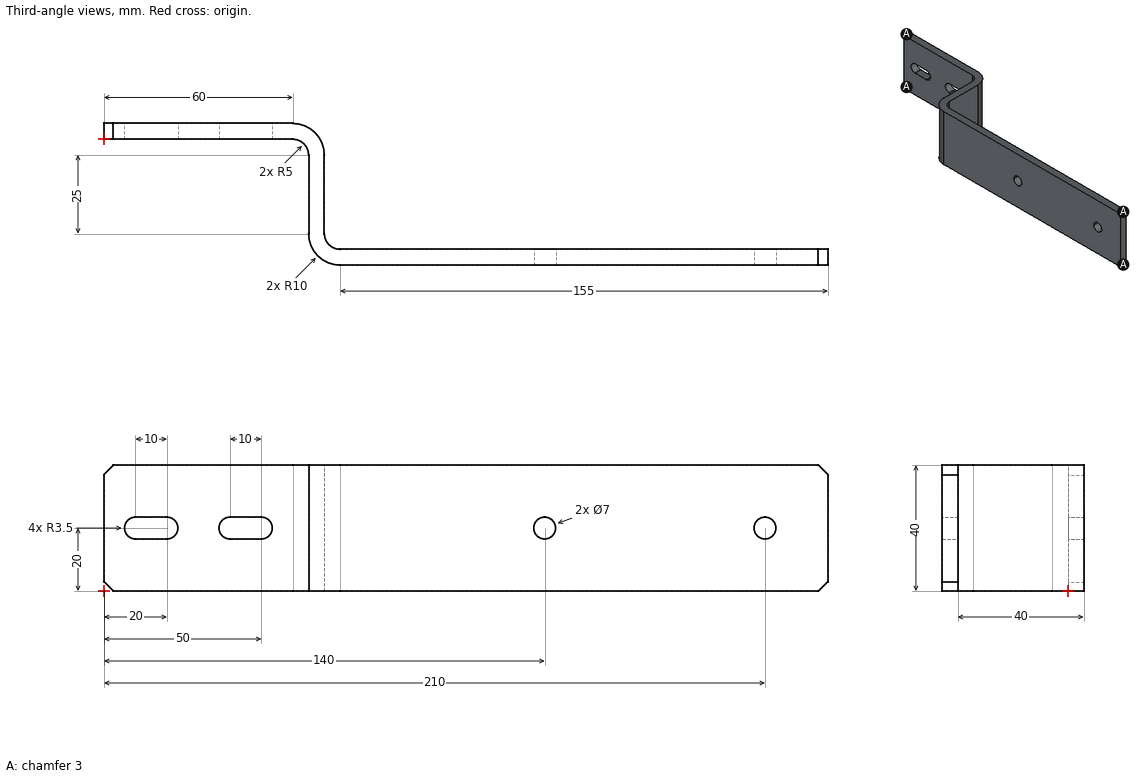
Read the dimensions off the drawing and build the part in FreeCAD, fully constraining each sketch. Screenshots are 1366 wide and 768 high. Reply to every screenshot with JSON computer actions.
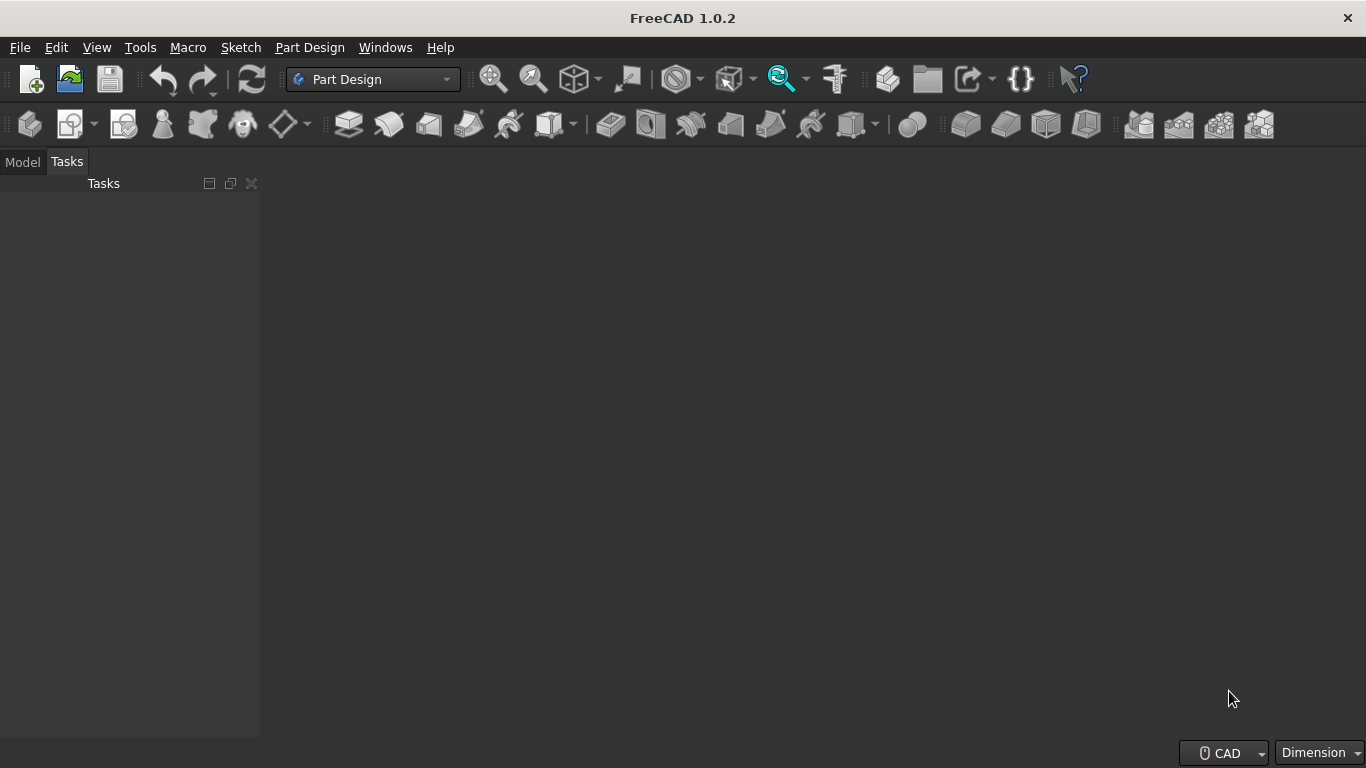
{"action": "left_click", "coordinate": [30, 80]}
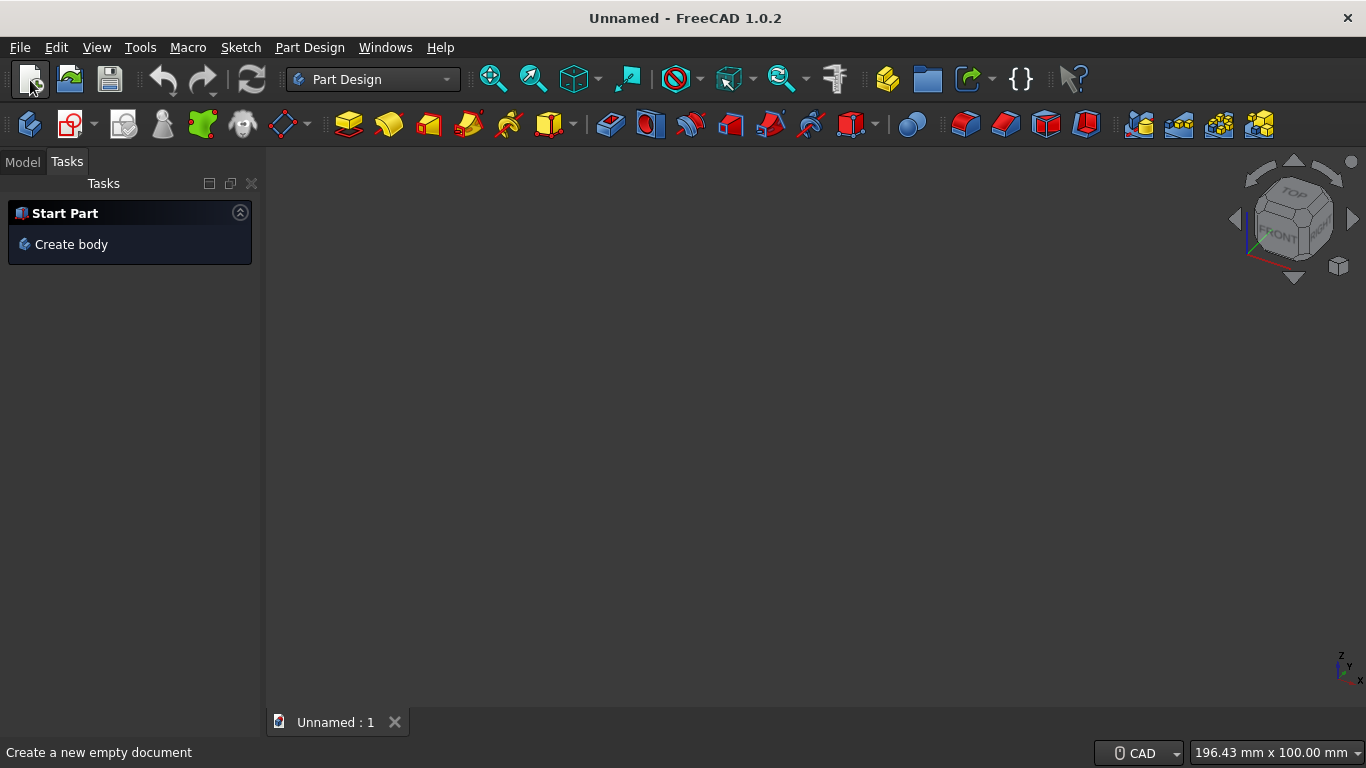
{"action": "left_click", "coordinate": [70, 124]}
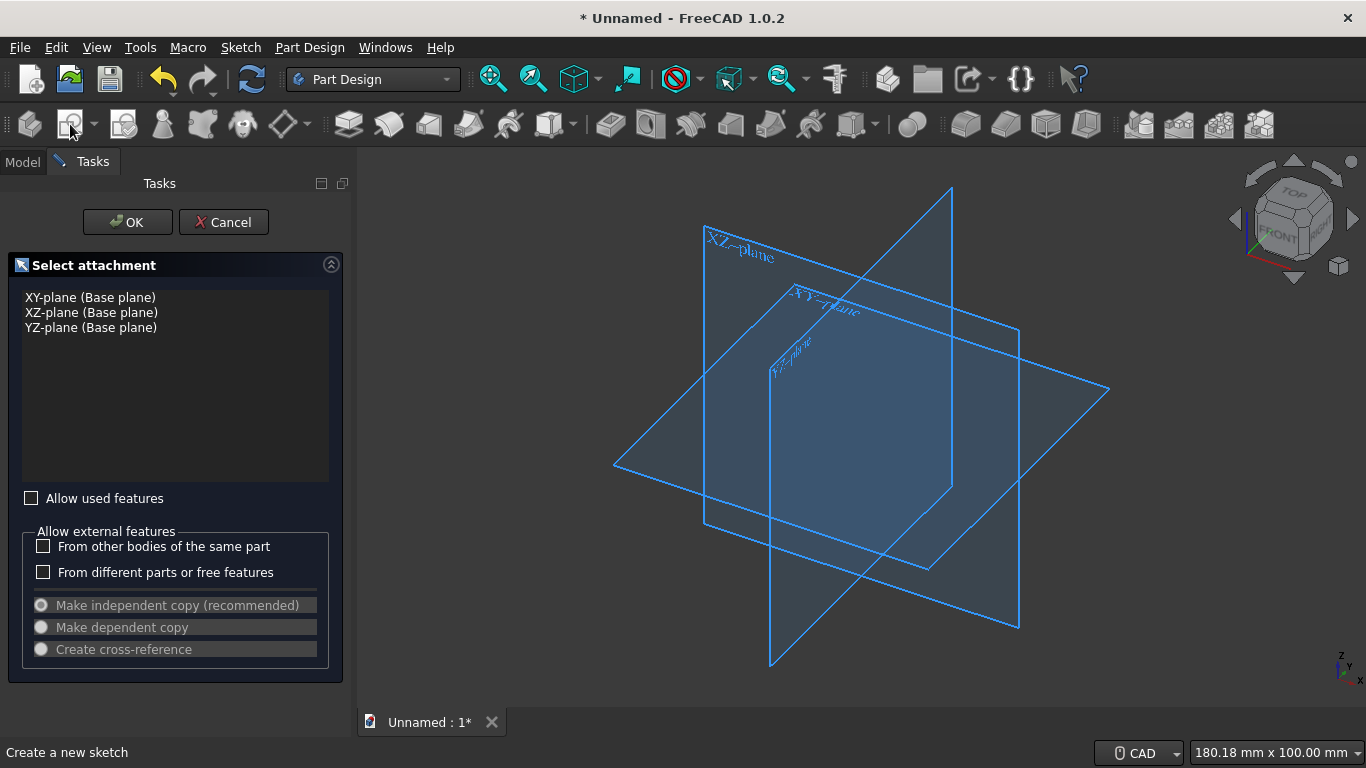
{"action": "left_click", "coordinate": [82, 298]}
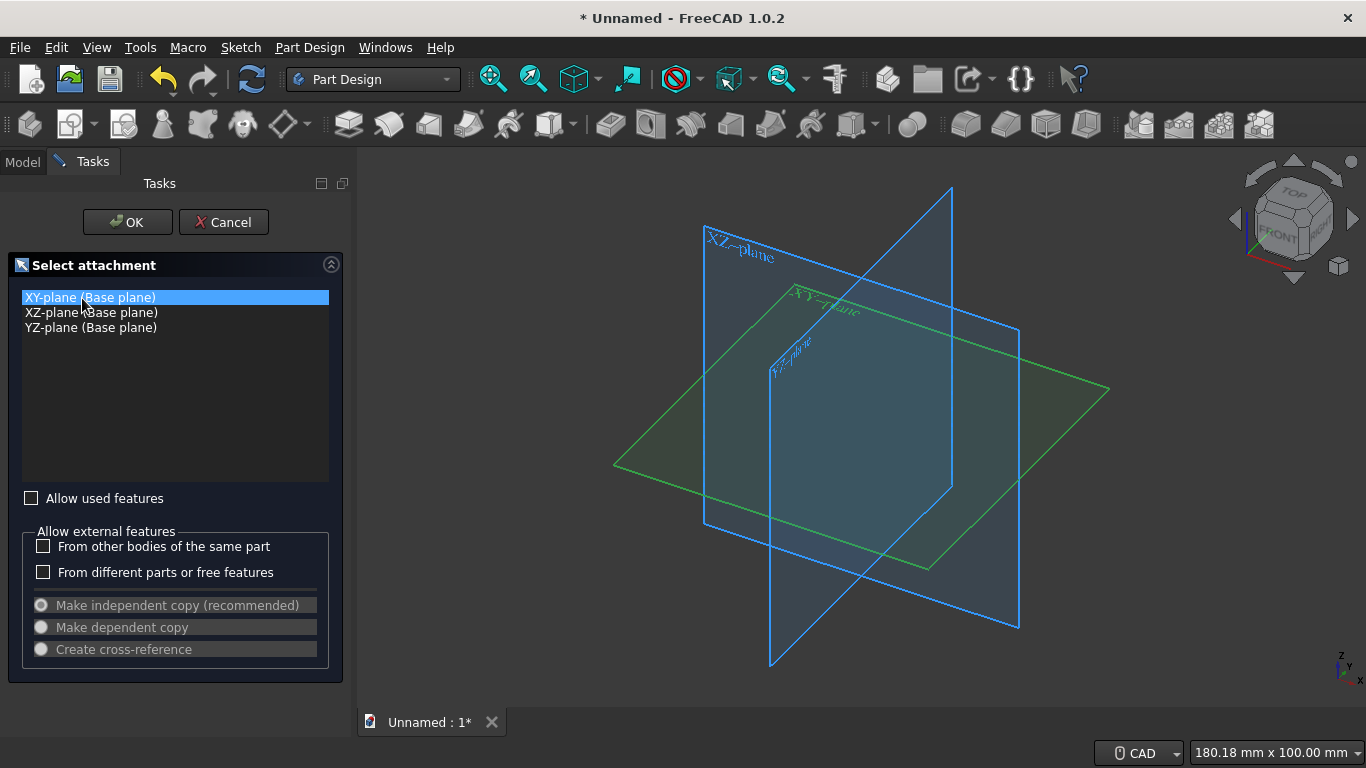
{"action": "left_click", "coordinate": [128, 222]}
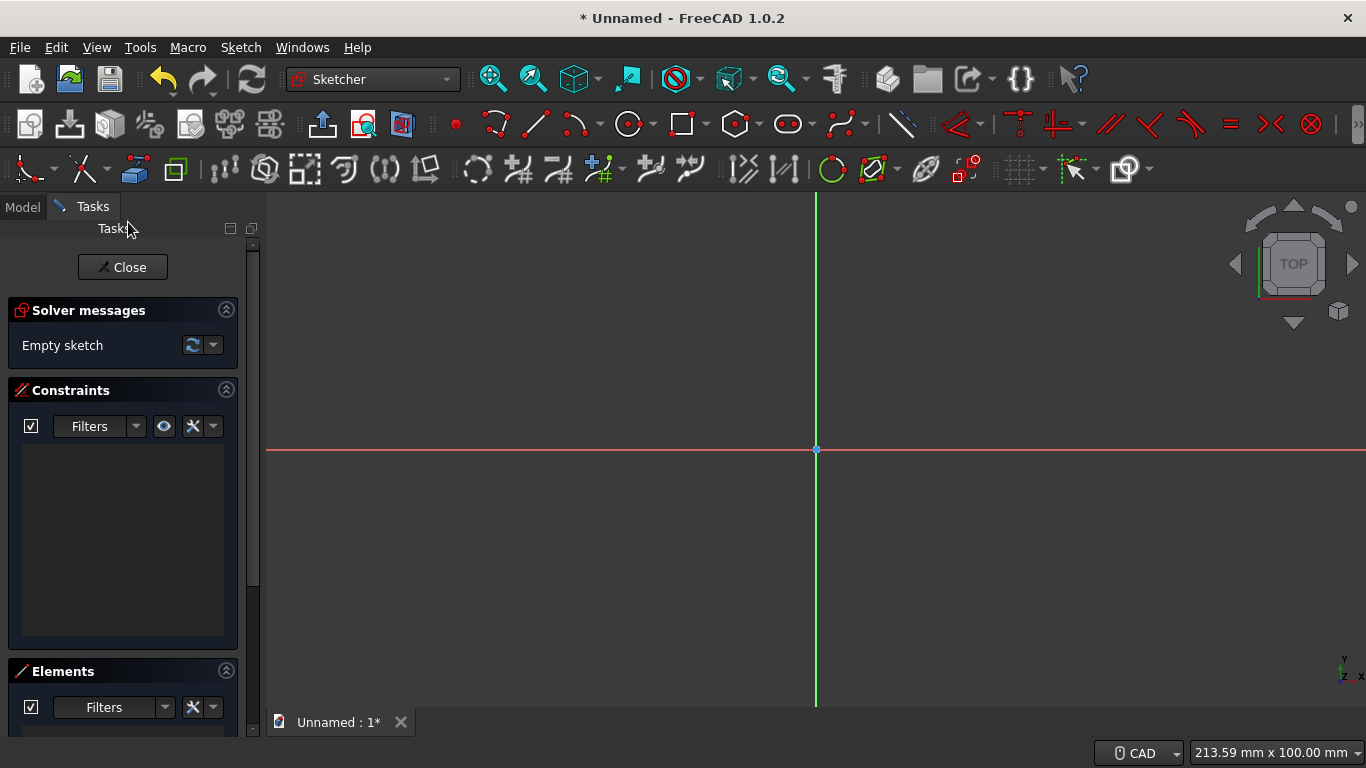
{"action": "scroll", "coordinate": [294, 376], "scroll_direction": "down", "scroll_amount": 4}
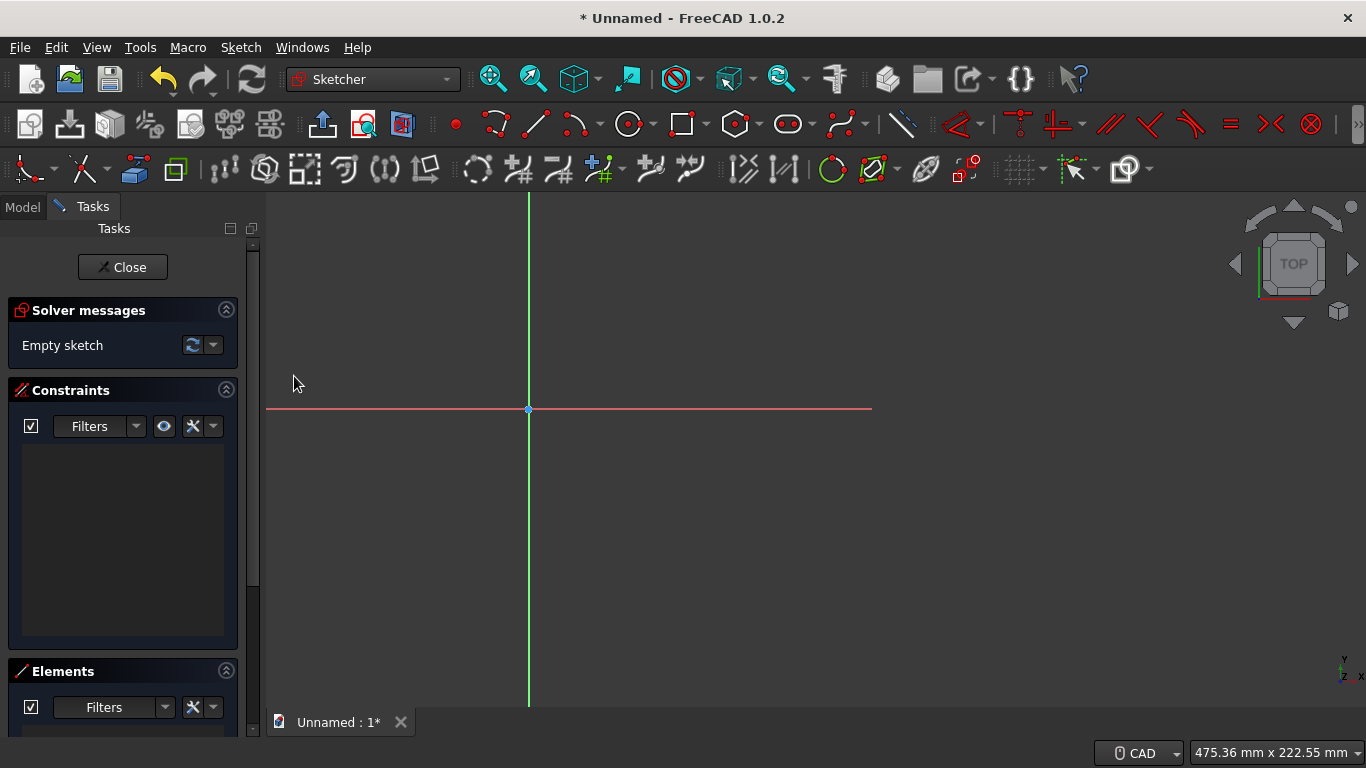
{"action": "left_click", "coordinate": [536, 124]}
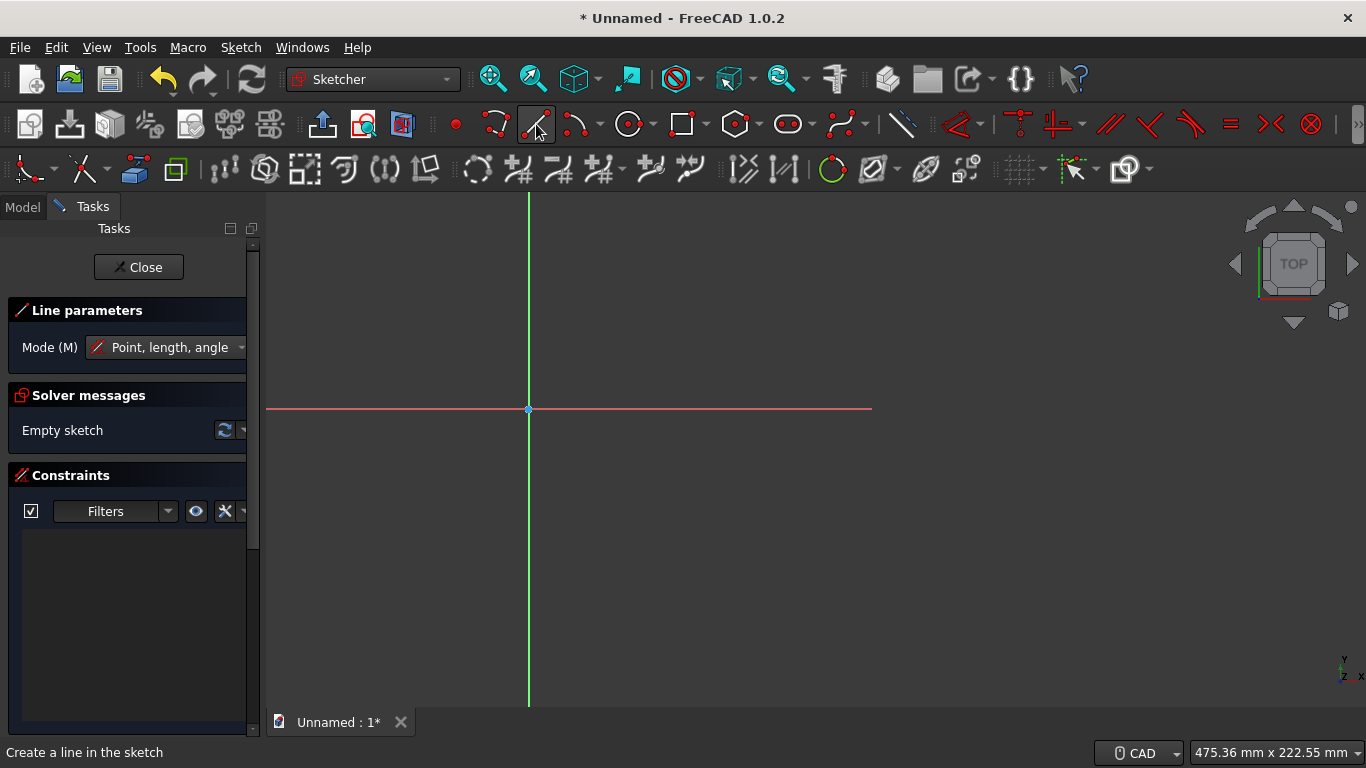
{"action": "scroll", "coordinate": [679, 421], "scroll_direction": "up", "scroll_amount": 2}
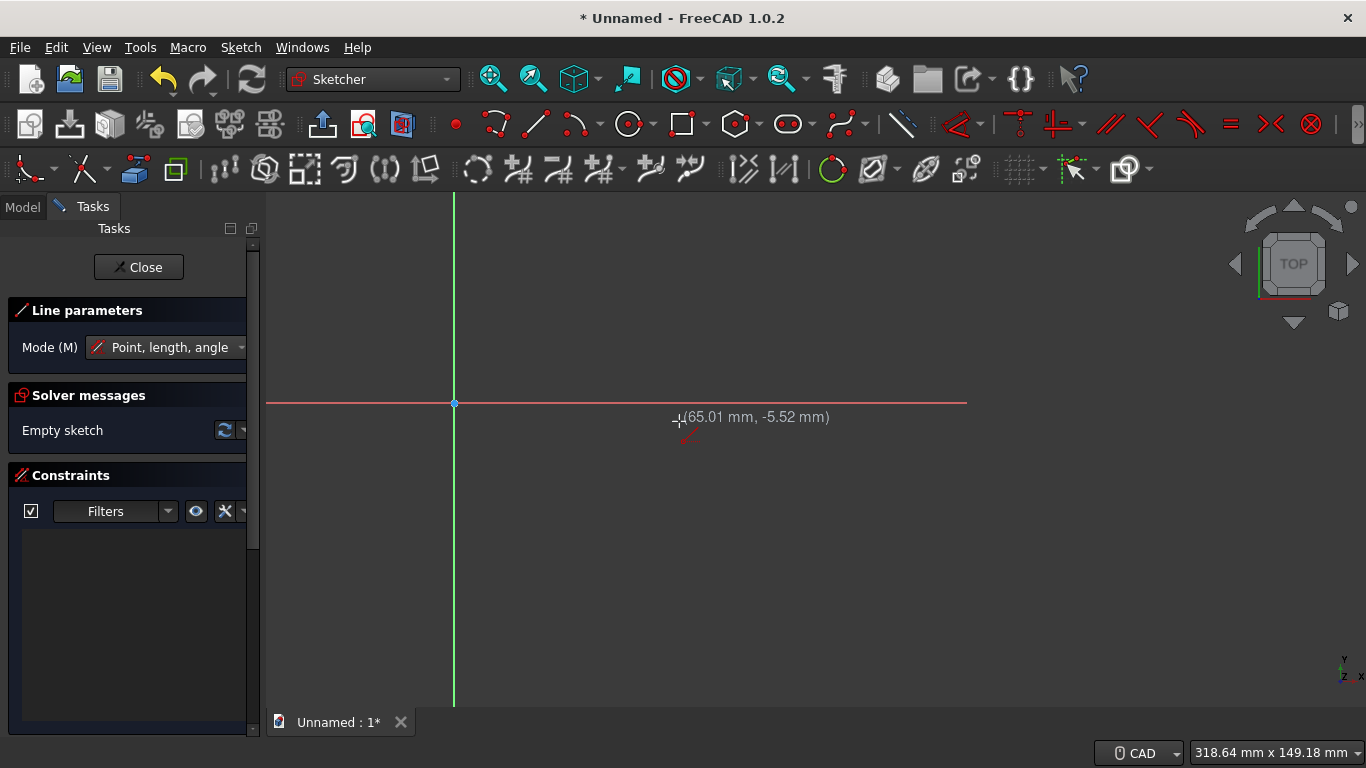
{"action": "left_click", "coordinate": [679, 420]}
{"action": "left_click", "coordinate": [679, 507]}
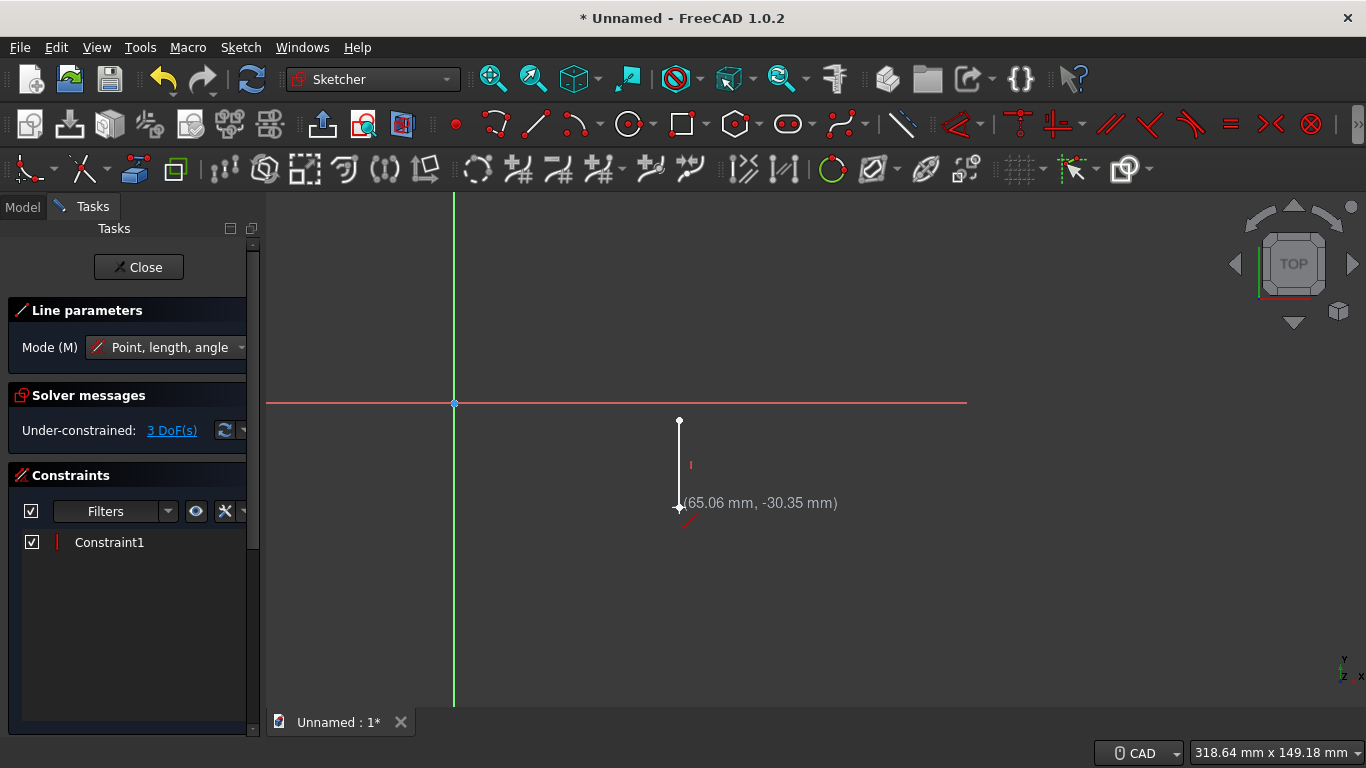
{"action": "left_click", "coordinate": [496, 124]}